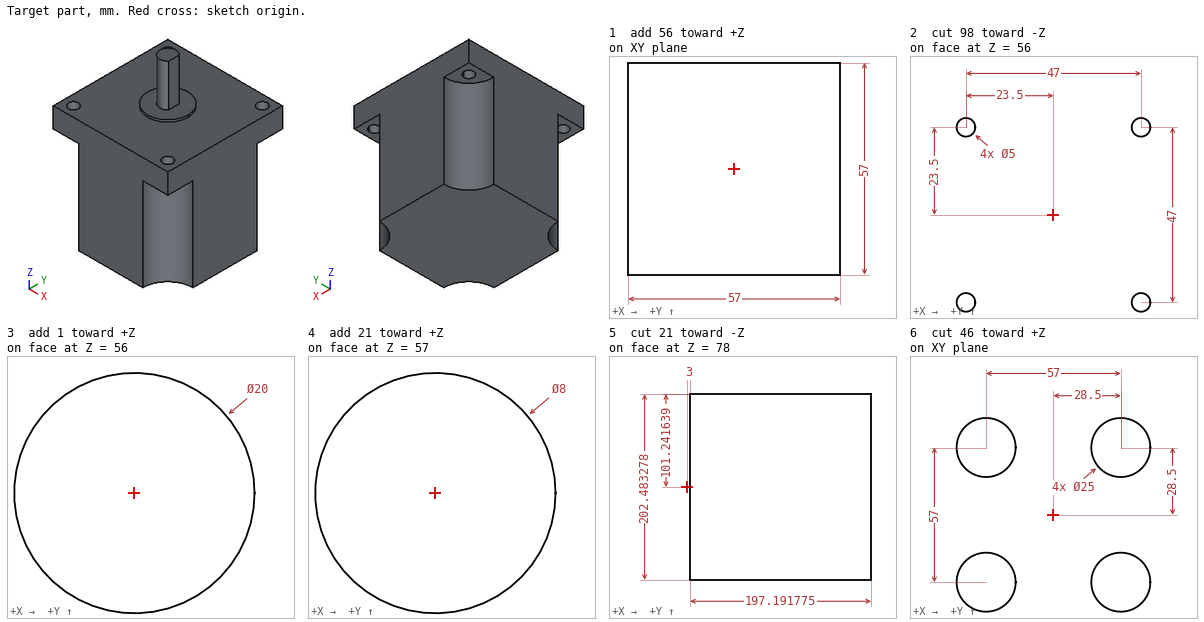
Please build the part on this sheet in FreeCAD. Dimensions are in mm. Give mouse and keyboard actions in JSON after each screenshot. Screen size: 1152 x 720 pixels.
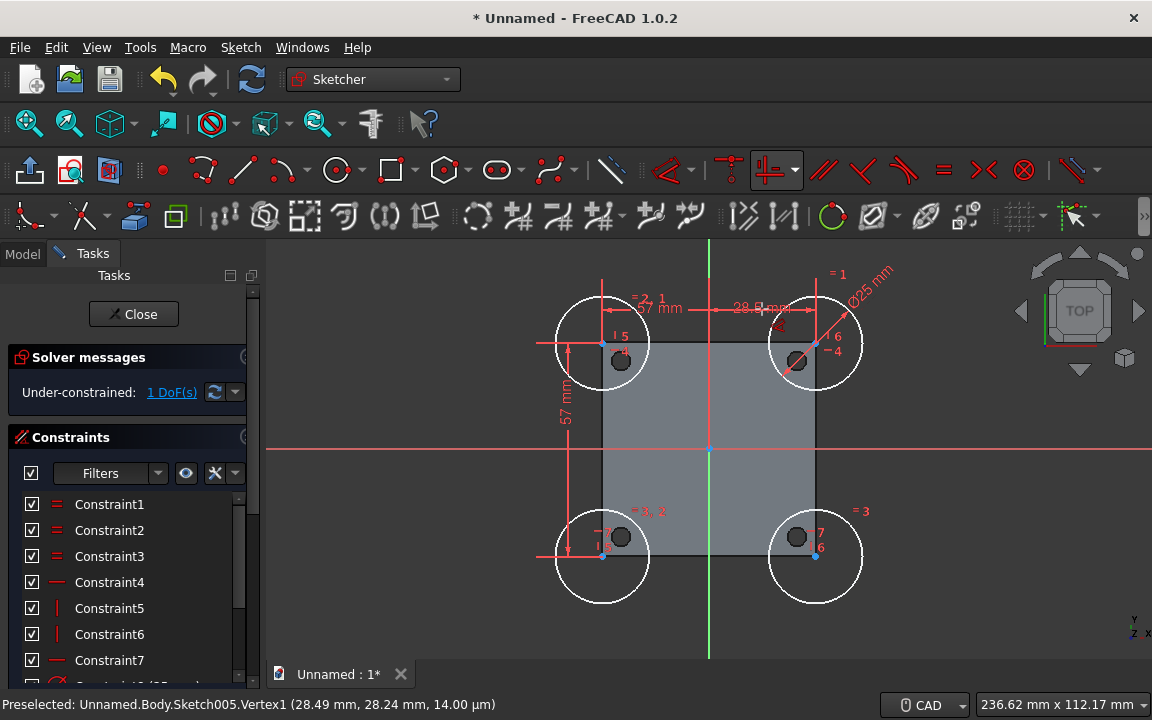
{"action": "left_click", "coordinate": [816, 343]}
{"action": "left_click", "coordinate": [850, 396]}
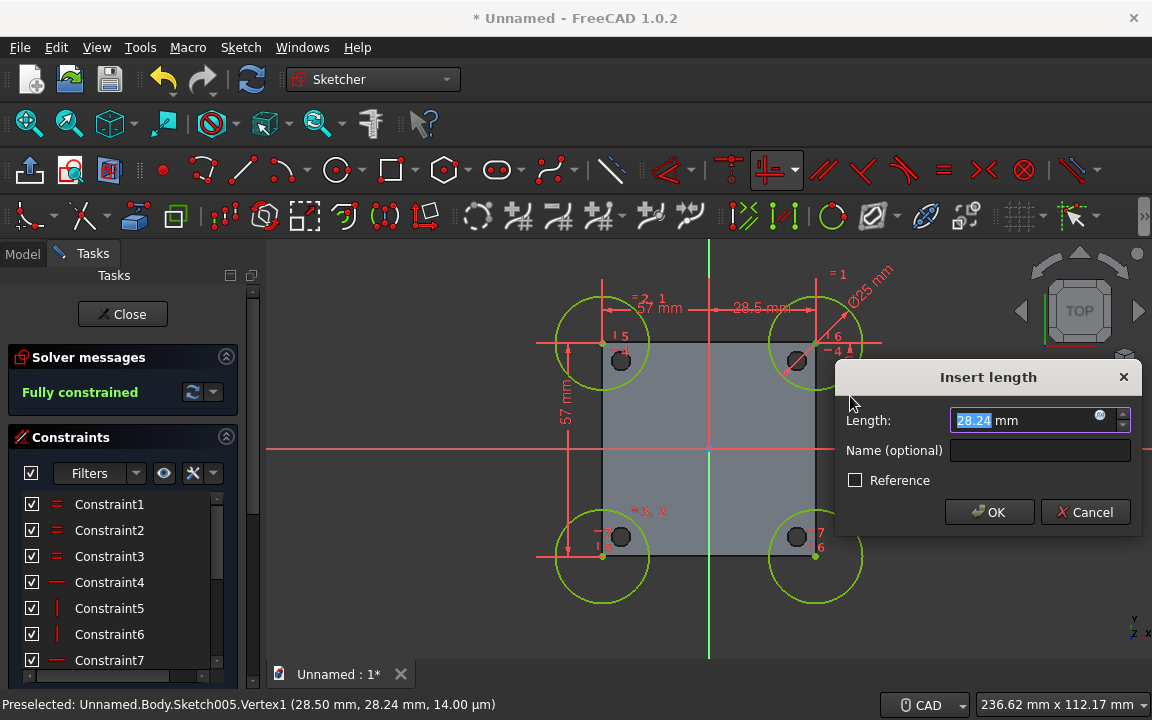
{"action": "type", "text": "28.5"}
{"action": "key", "text": "Return"}
{"action": "key", "text": "Escape"}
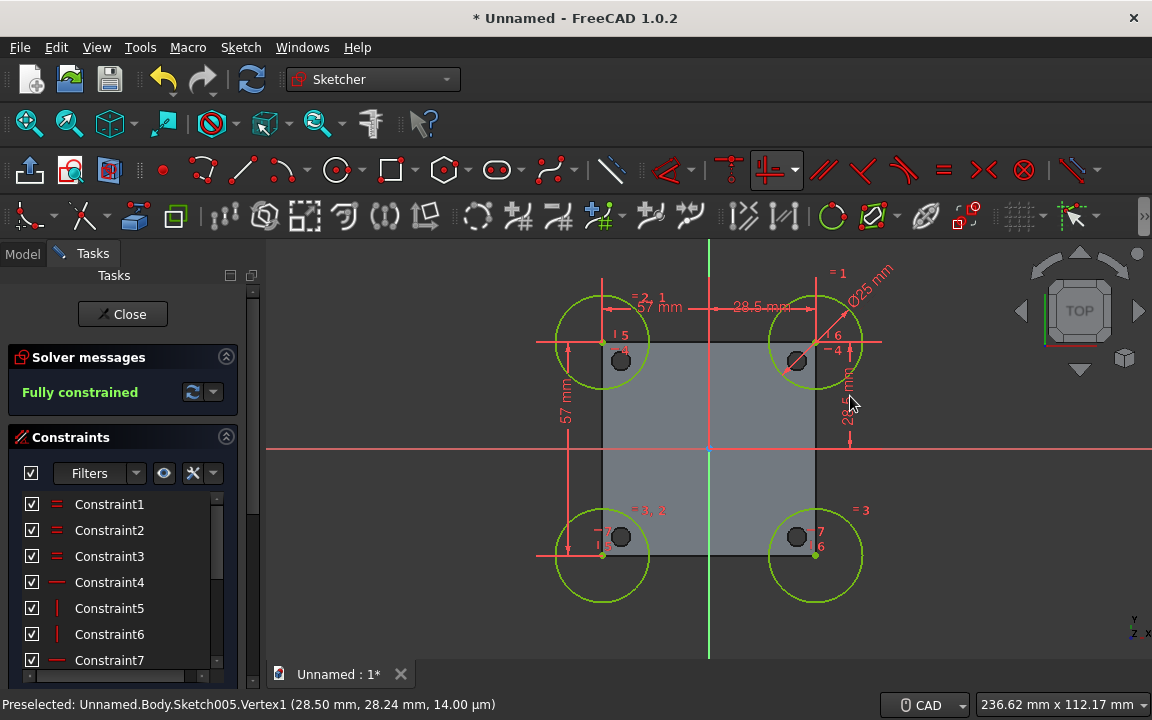
{"action": "left_click", "coordinate": [123, 314]}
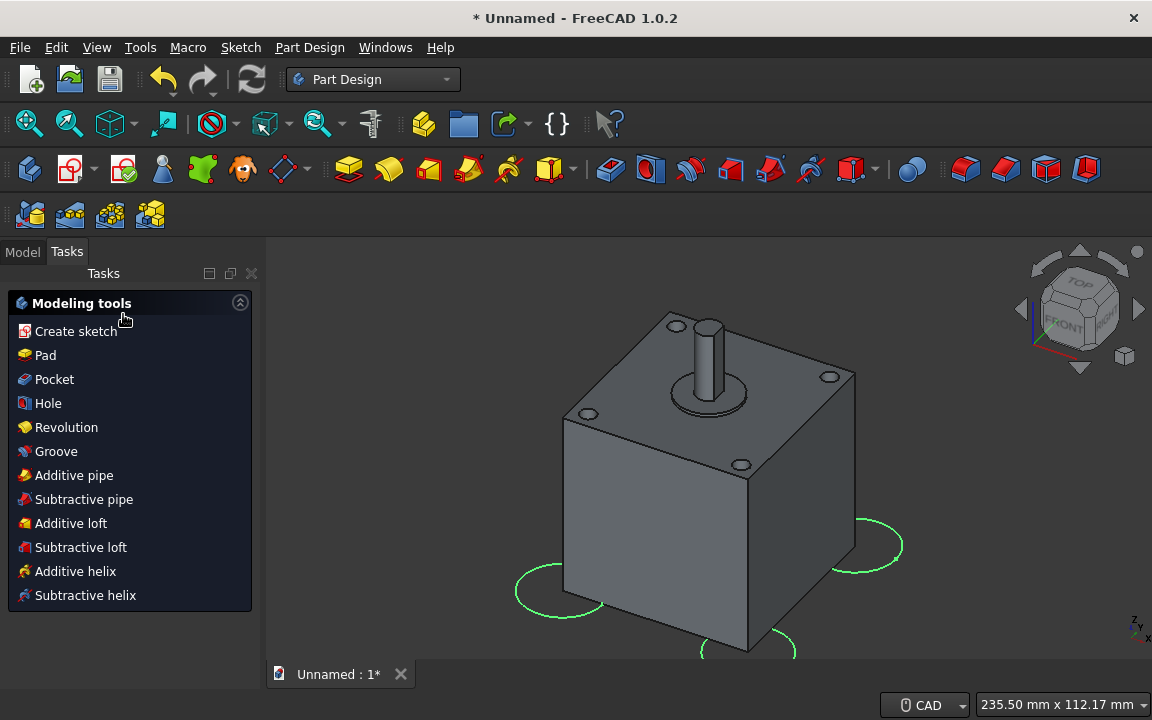
{"action": "left_click", "coordinate": [612, 170]}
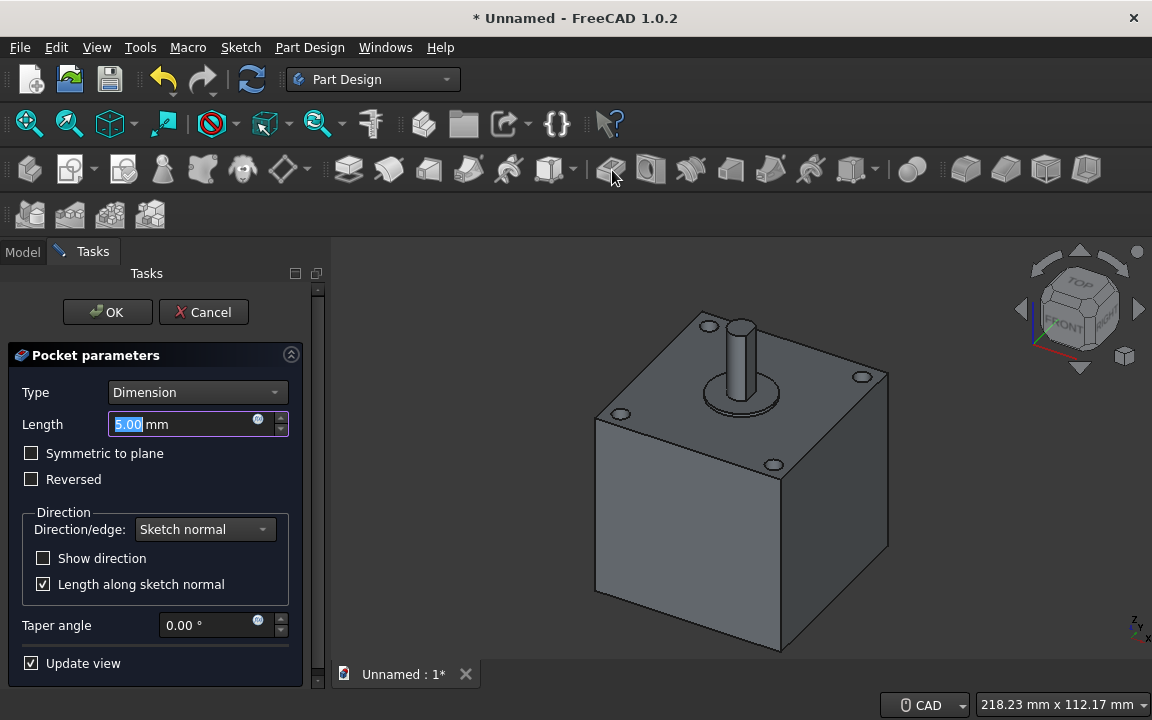
{"action": "type", "text": "46"}
{"action": "key", "text": "Tab"}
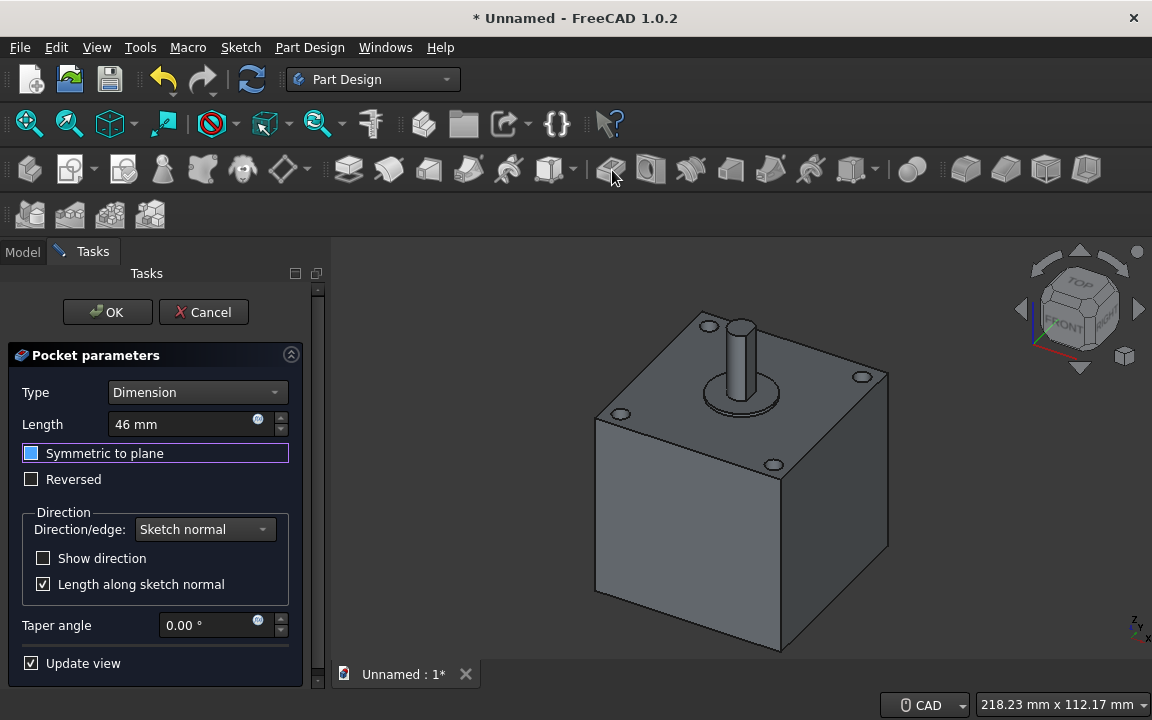
{"action": "left_click", "coordinate": [30, 479]}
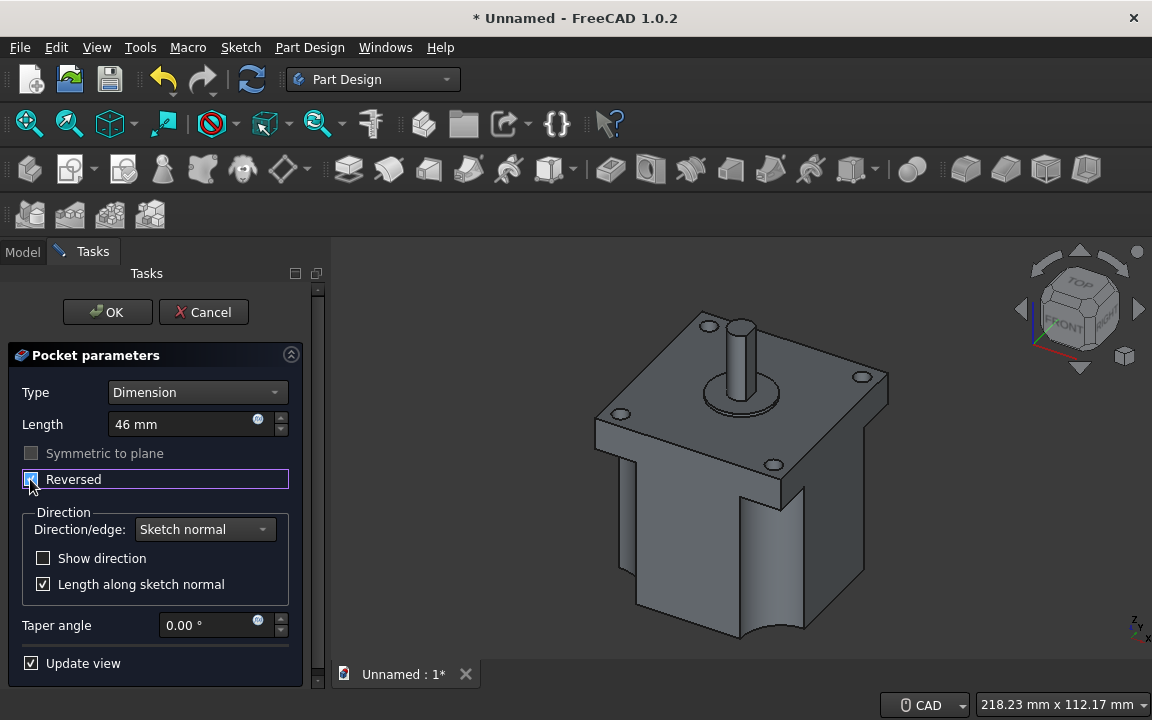
{"action": "left_click", "coordinate": [108, 312]}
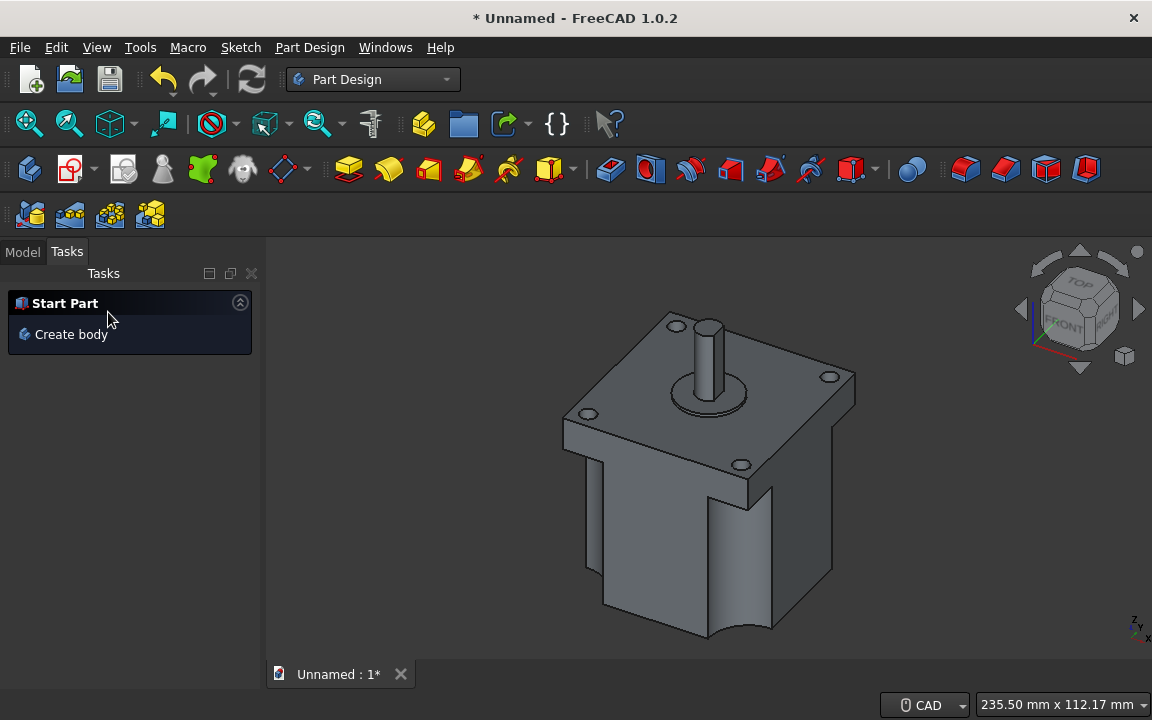
{"action": "key", "text": "0"}